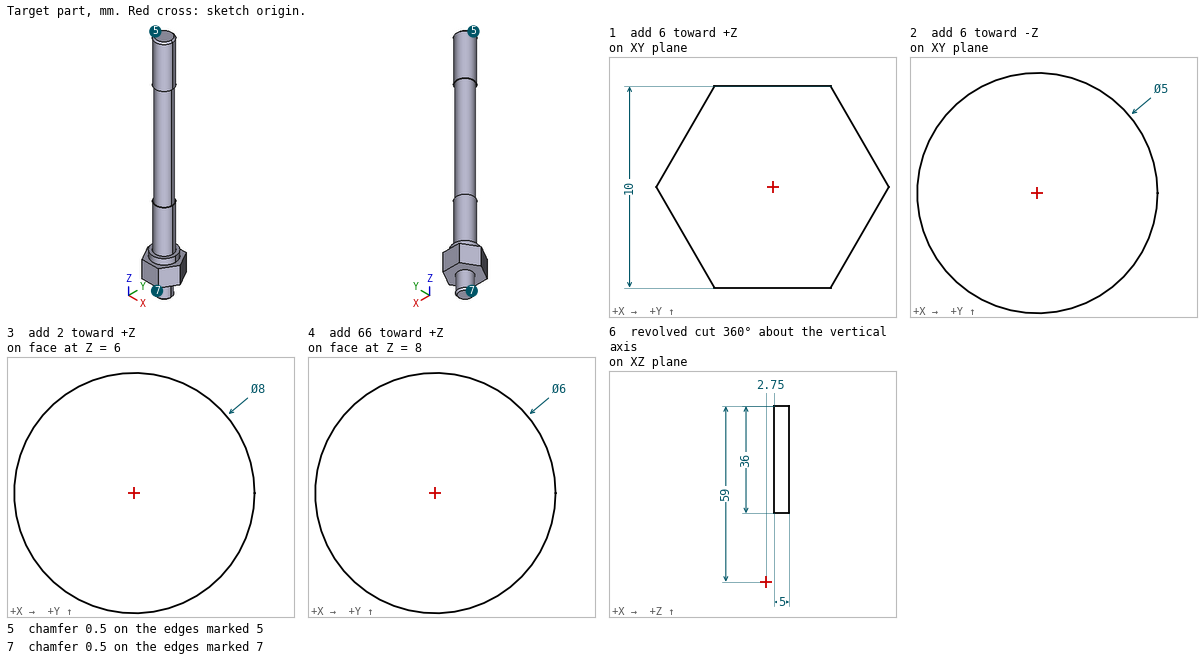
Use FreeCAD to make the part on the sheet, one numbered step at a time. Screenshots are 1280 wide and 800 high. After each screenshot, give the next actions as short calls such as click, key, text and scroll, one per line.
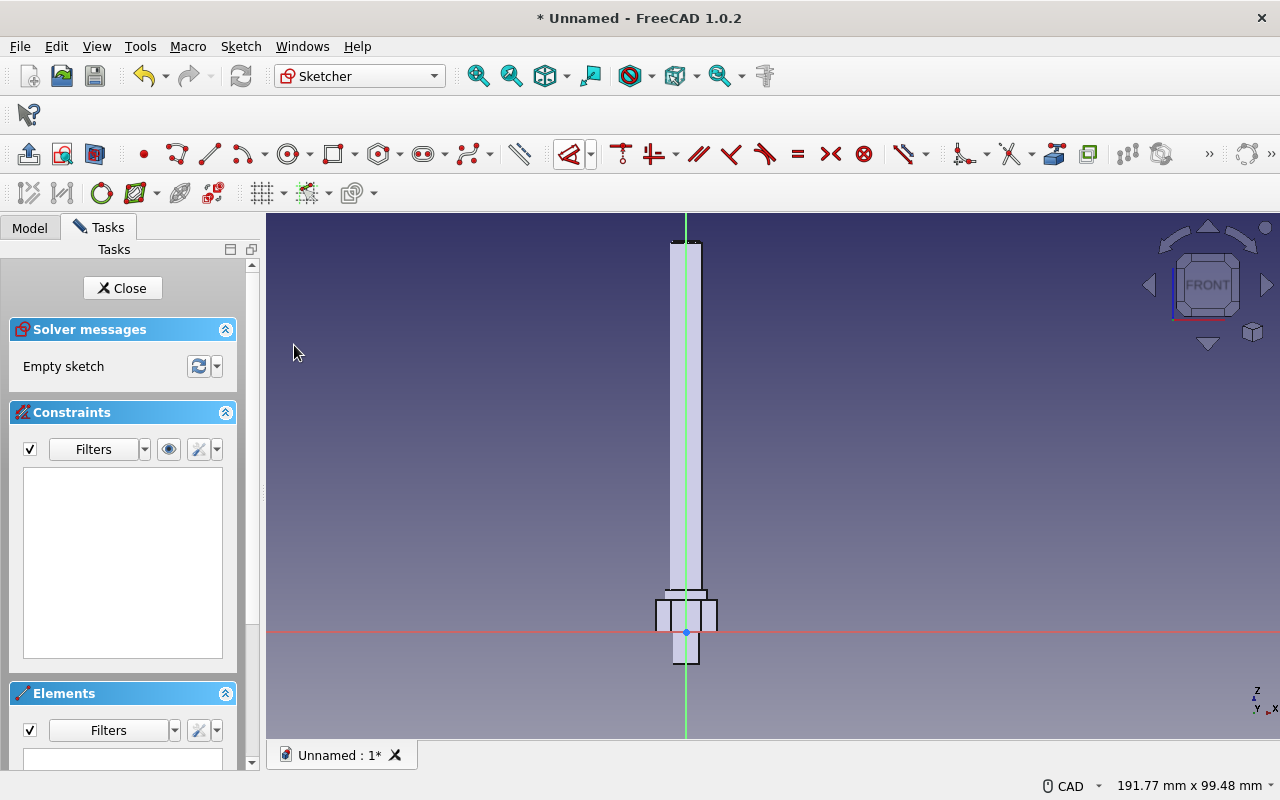
click(332, 154)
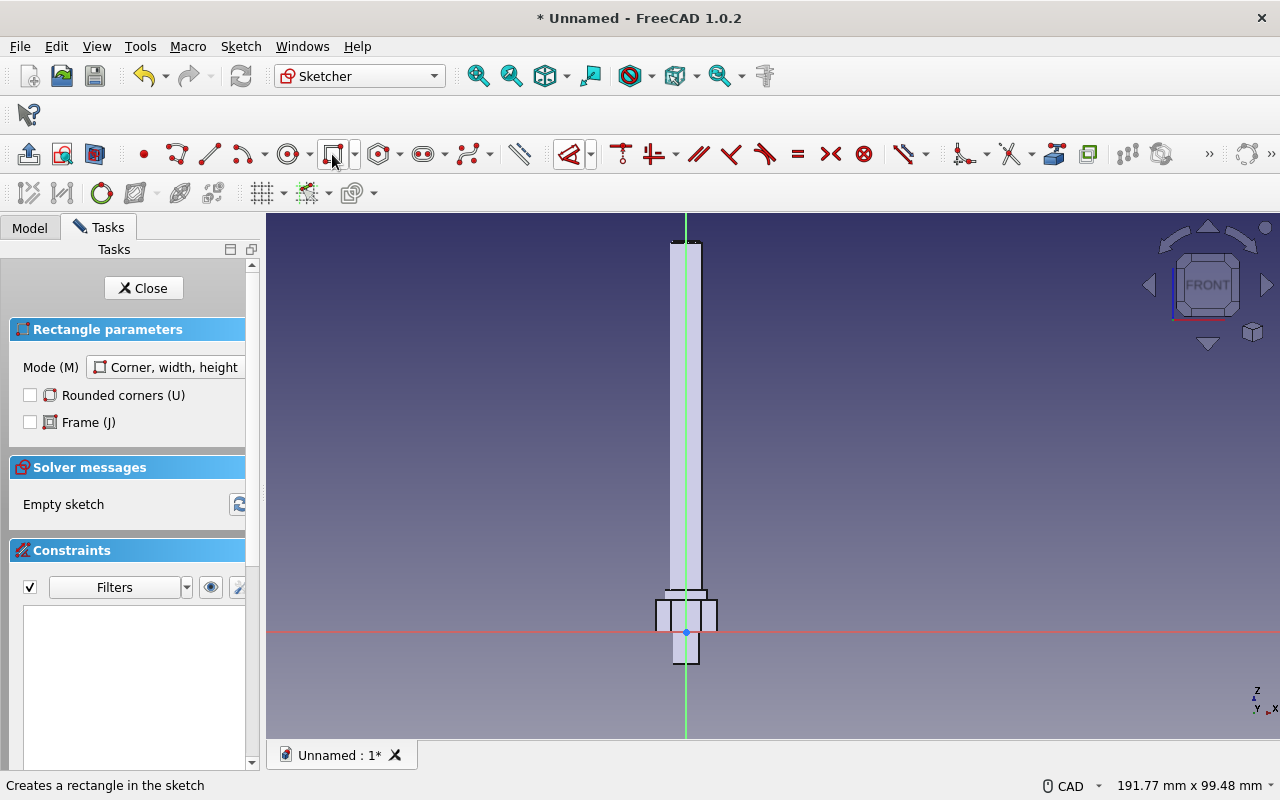
click(701, 320)
click(727, 510)
key(Escape)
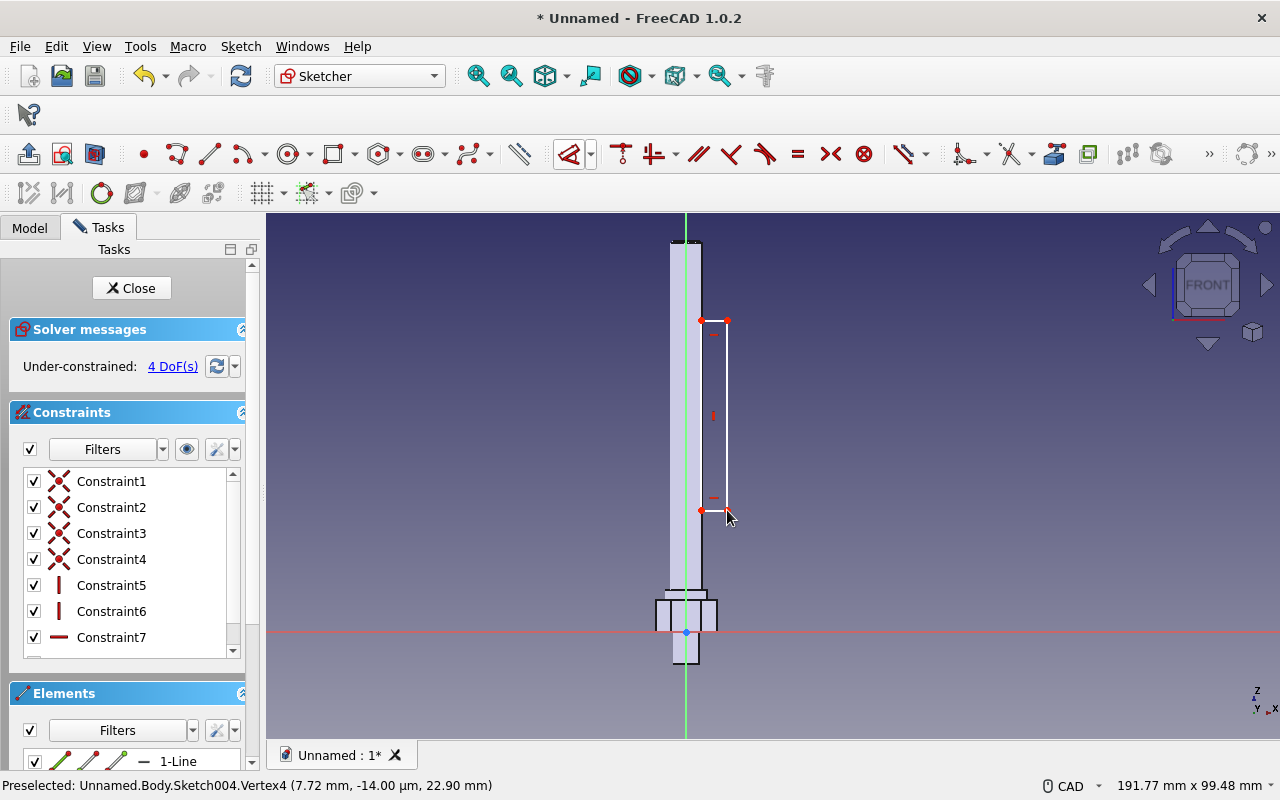
scroll(711, 511, up, 3)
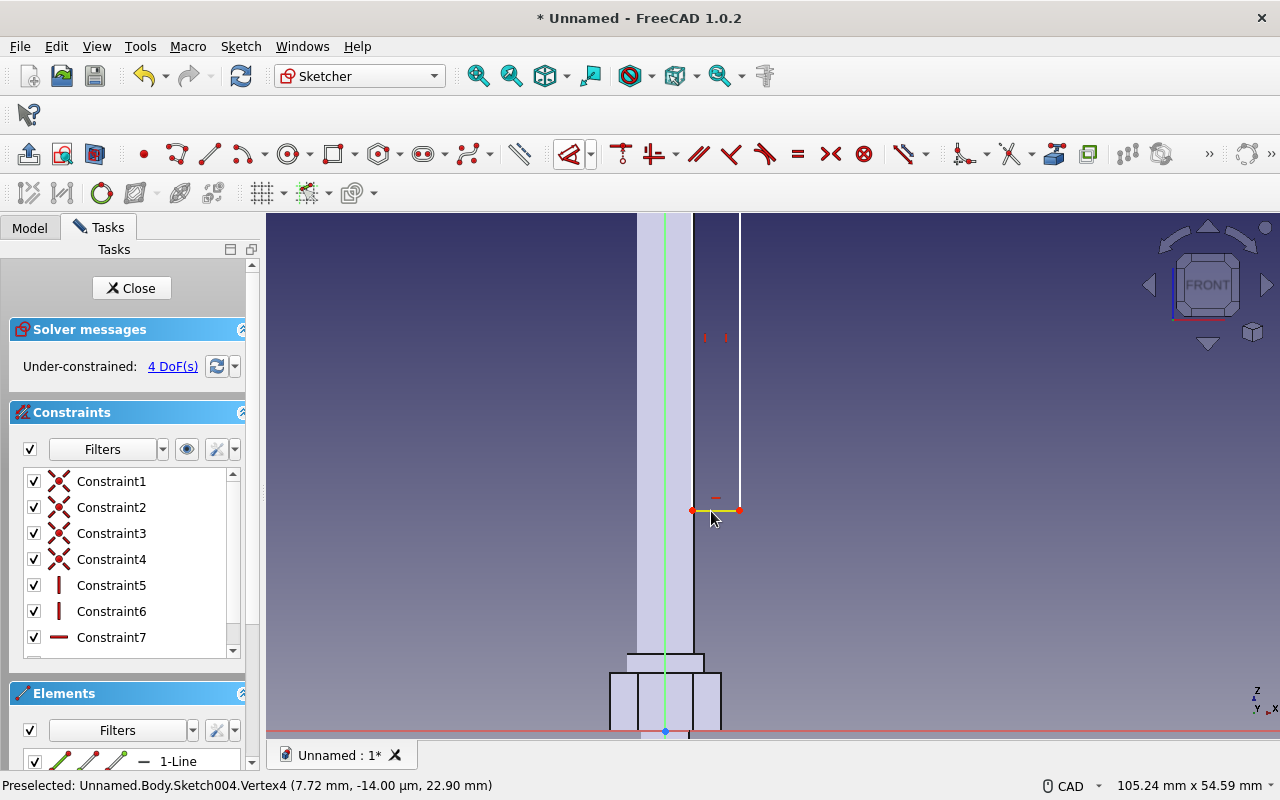
click(711, 511)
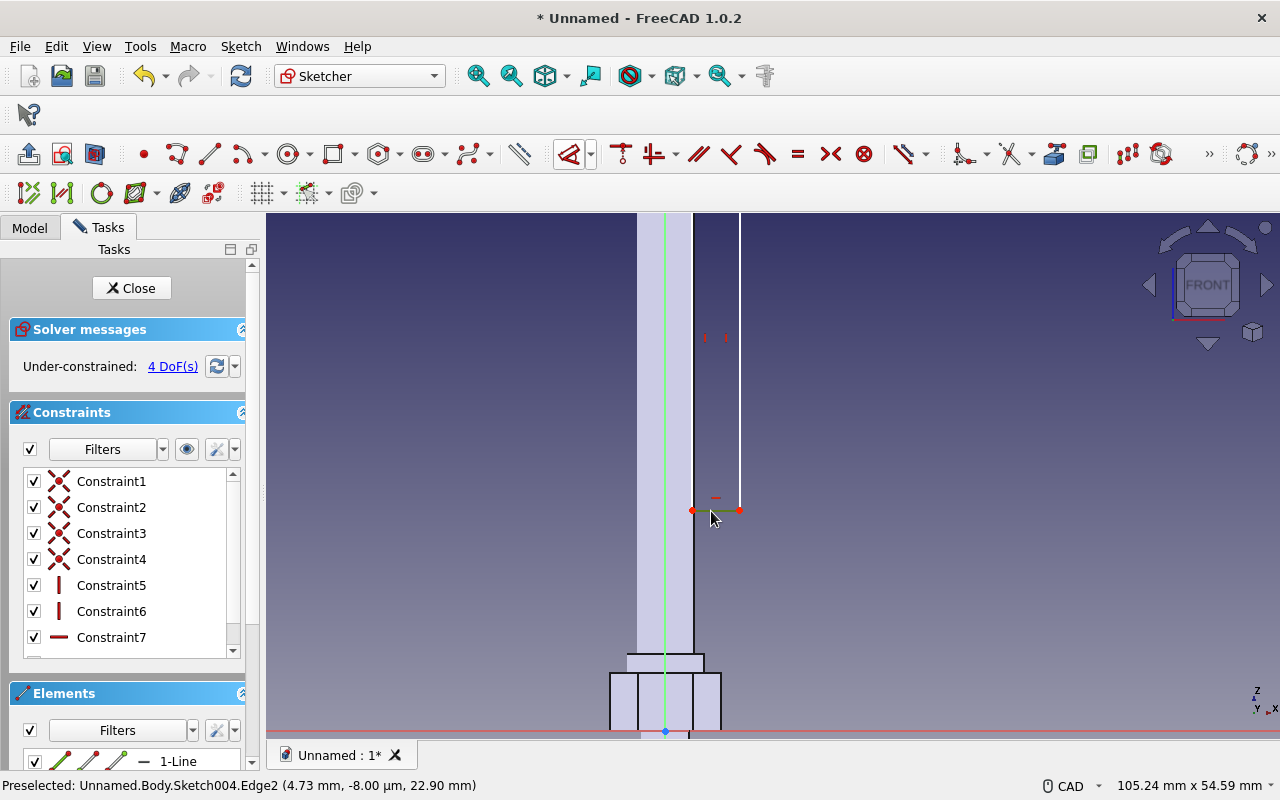
click(590, 154)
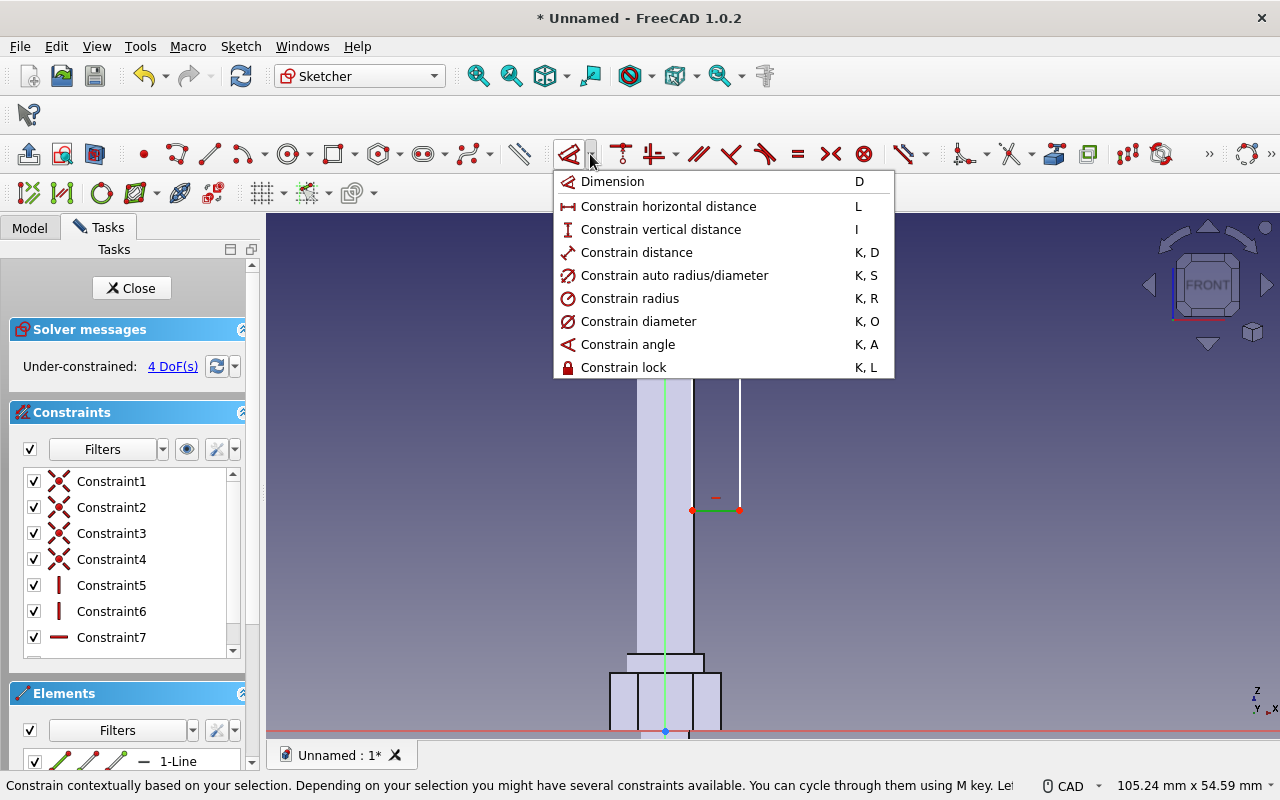
click(724, 206)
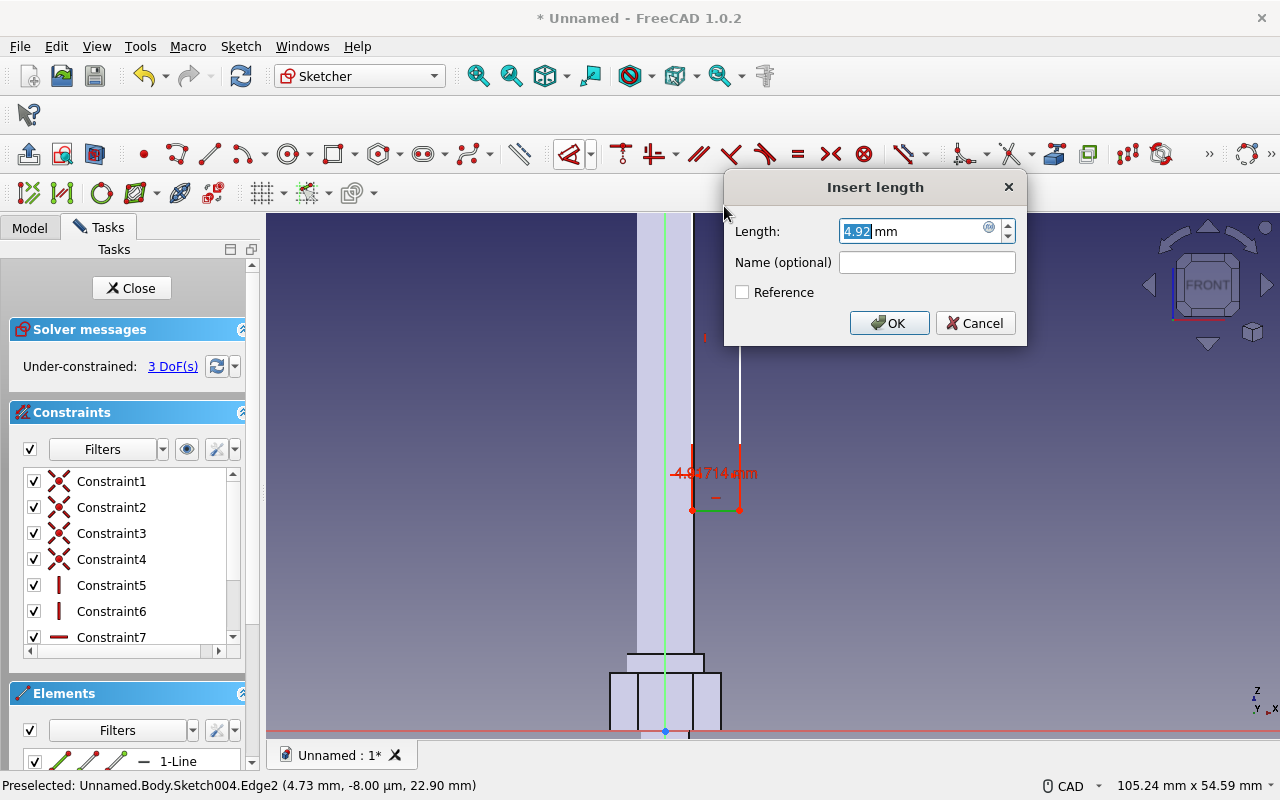
text(5)
key(Return)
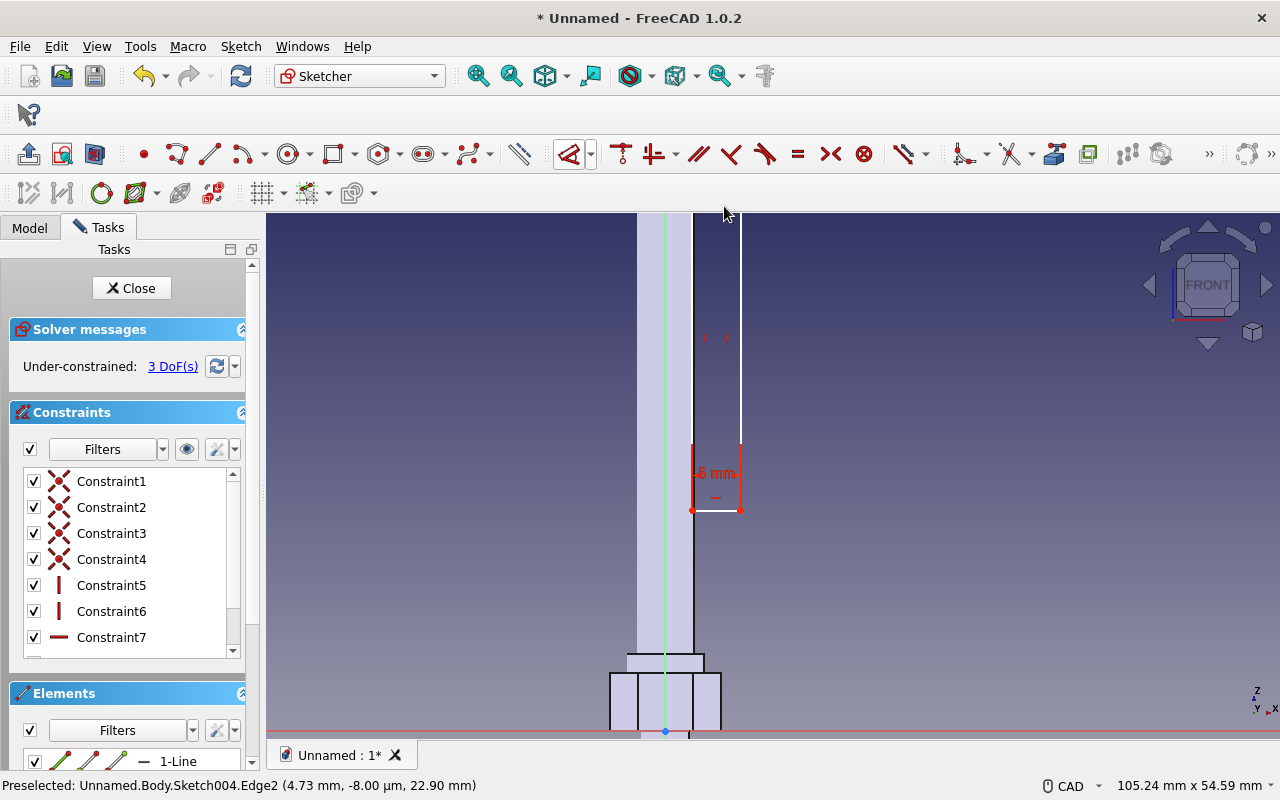
click(692, 268)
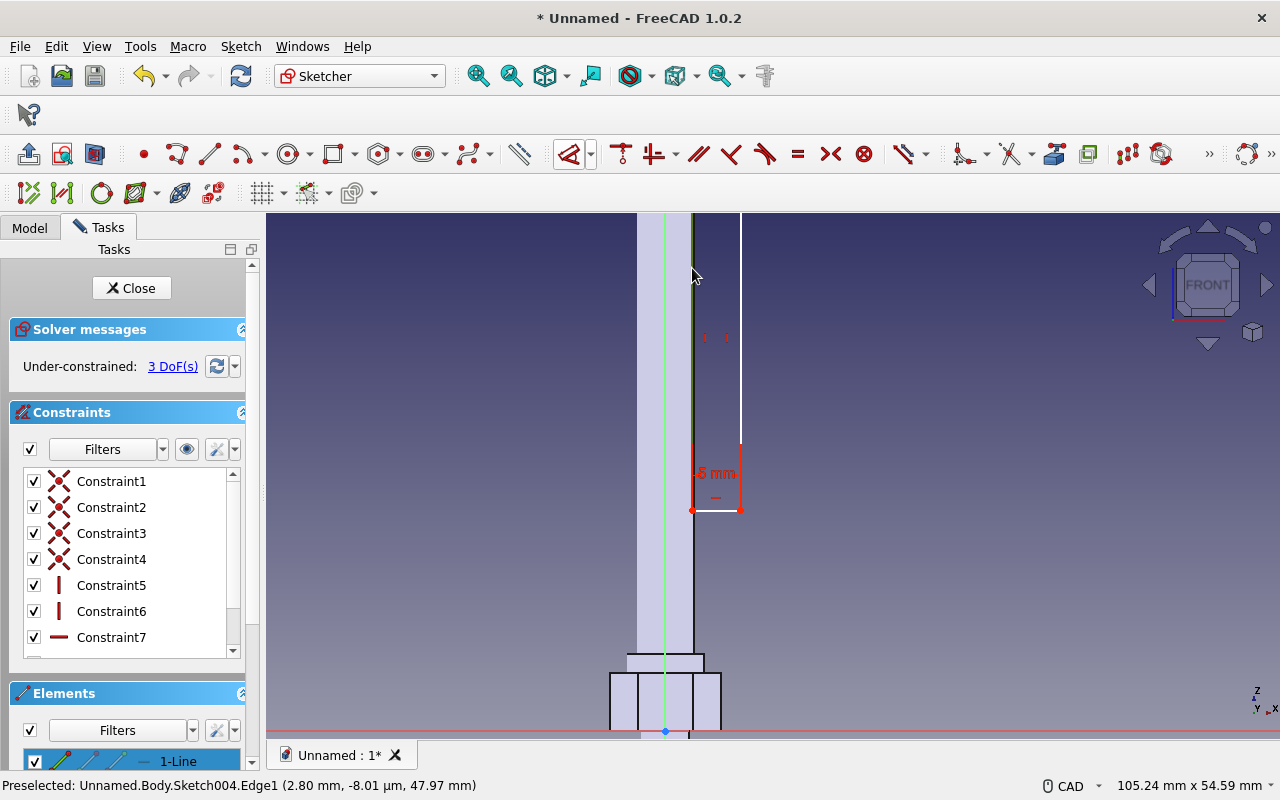
click(590, 154)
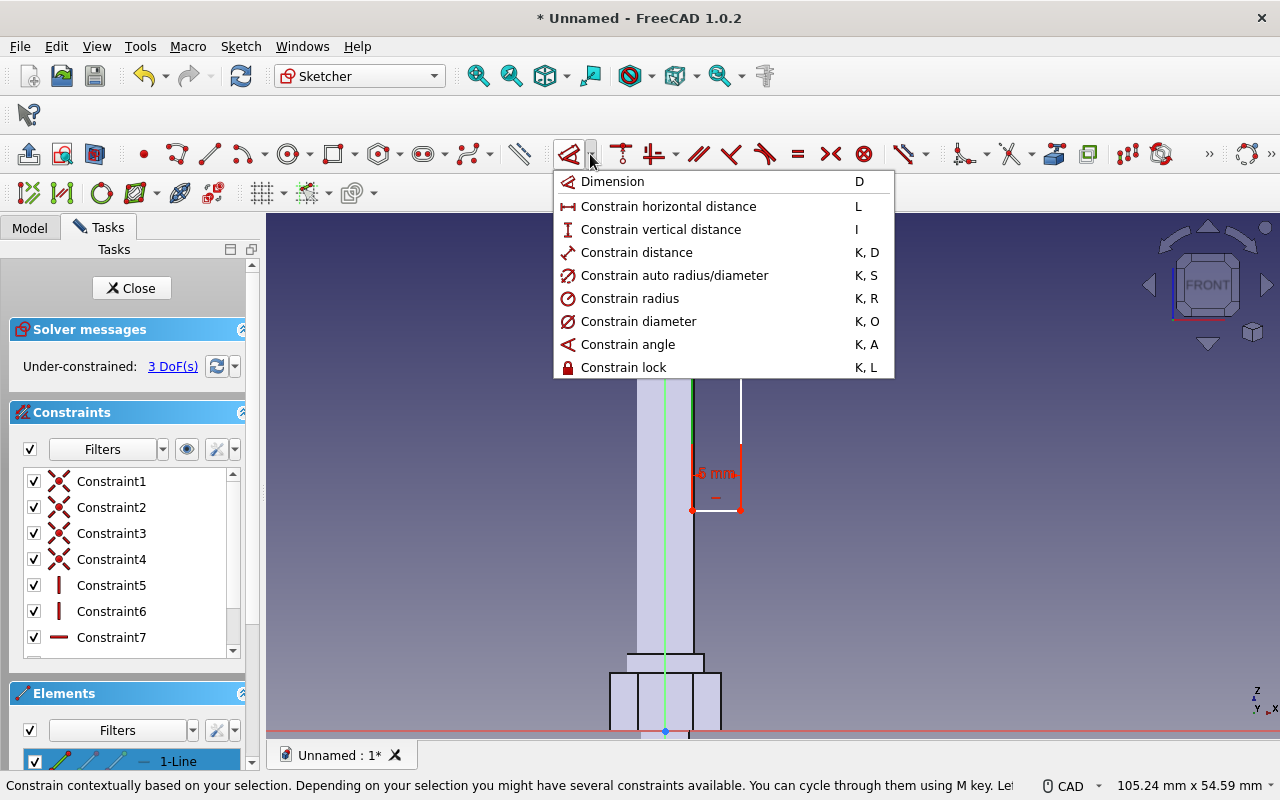
click(724, 230)